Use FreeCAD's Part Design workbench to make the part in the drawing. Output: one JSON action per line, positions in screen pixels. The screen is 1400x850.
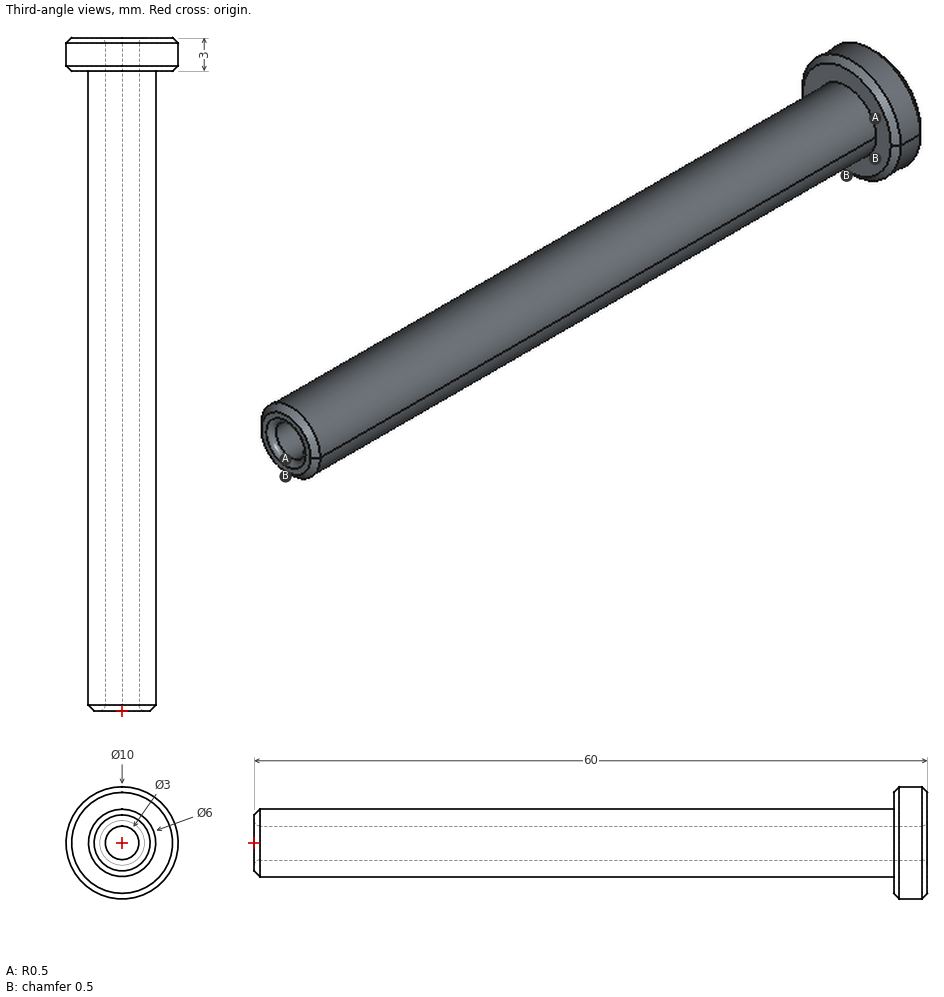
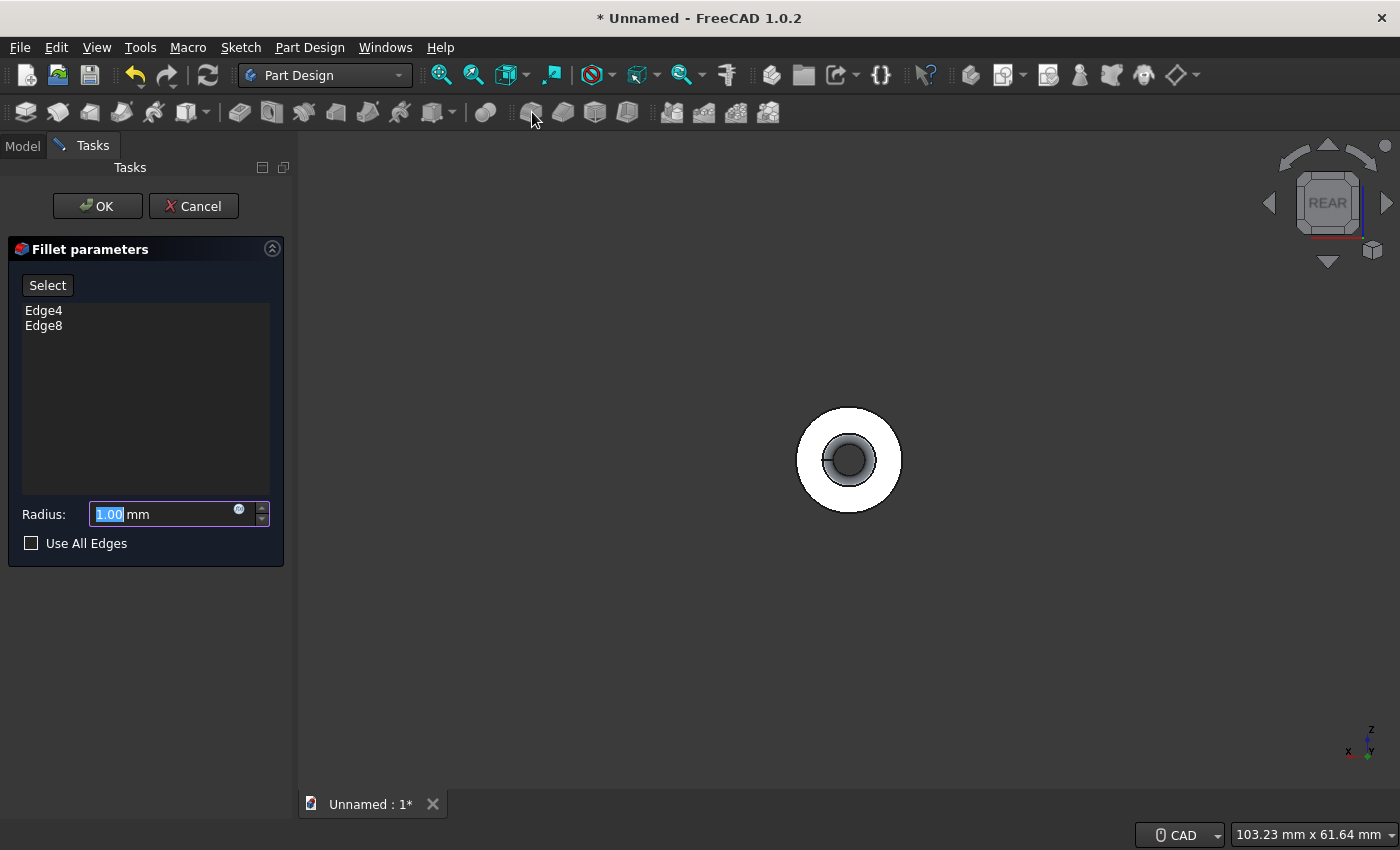
{"action": "type", "text": "0.5"}
{"action": "key", "text": "Tab"}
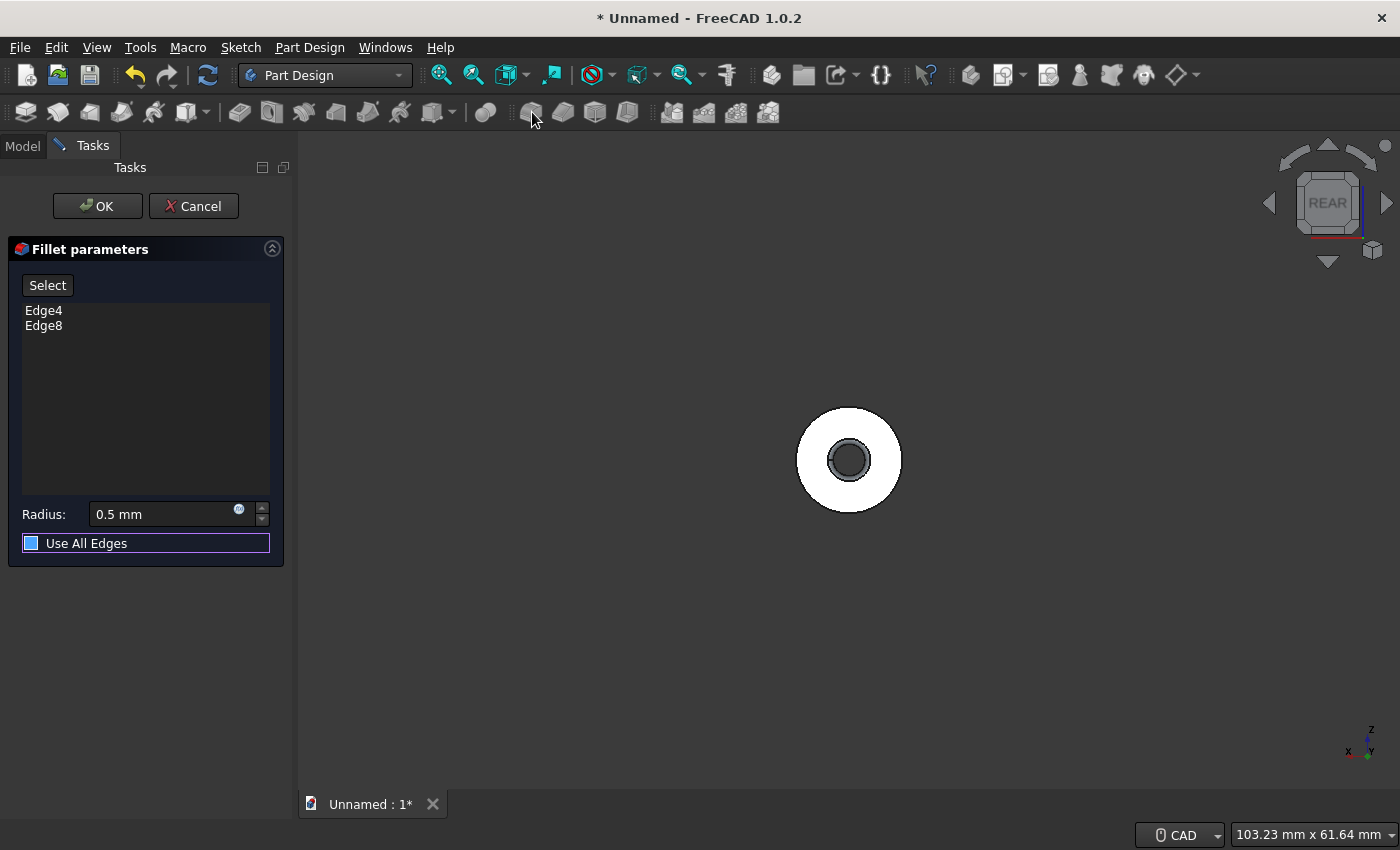
{"action": "left_click", "coordinate": [98, 206]}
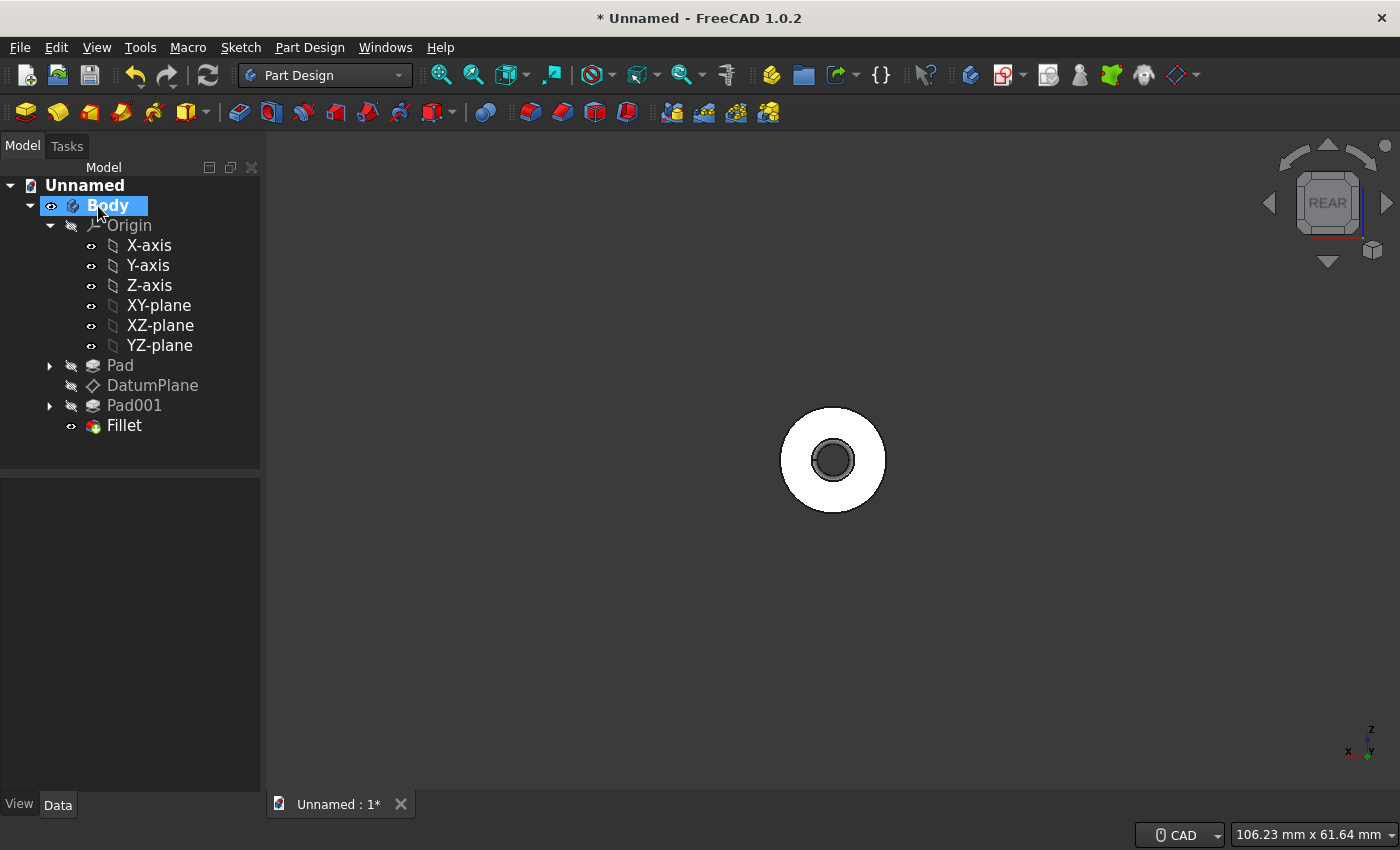
{"action": "left_click", "coordinate": [442, 76]}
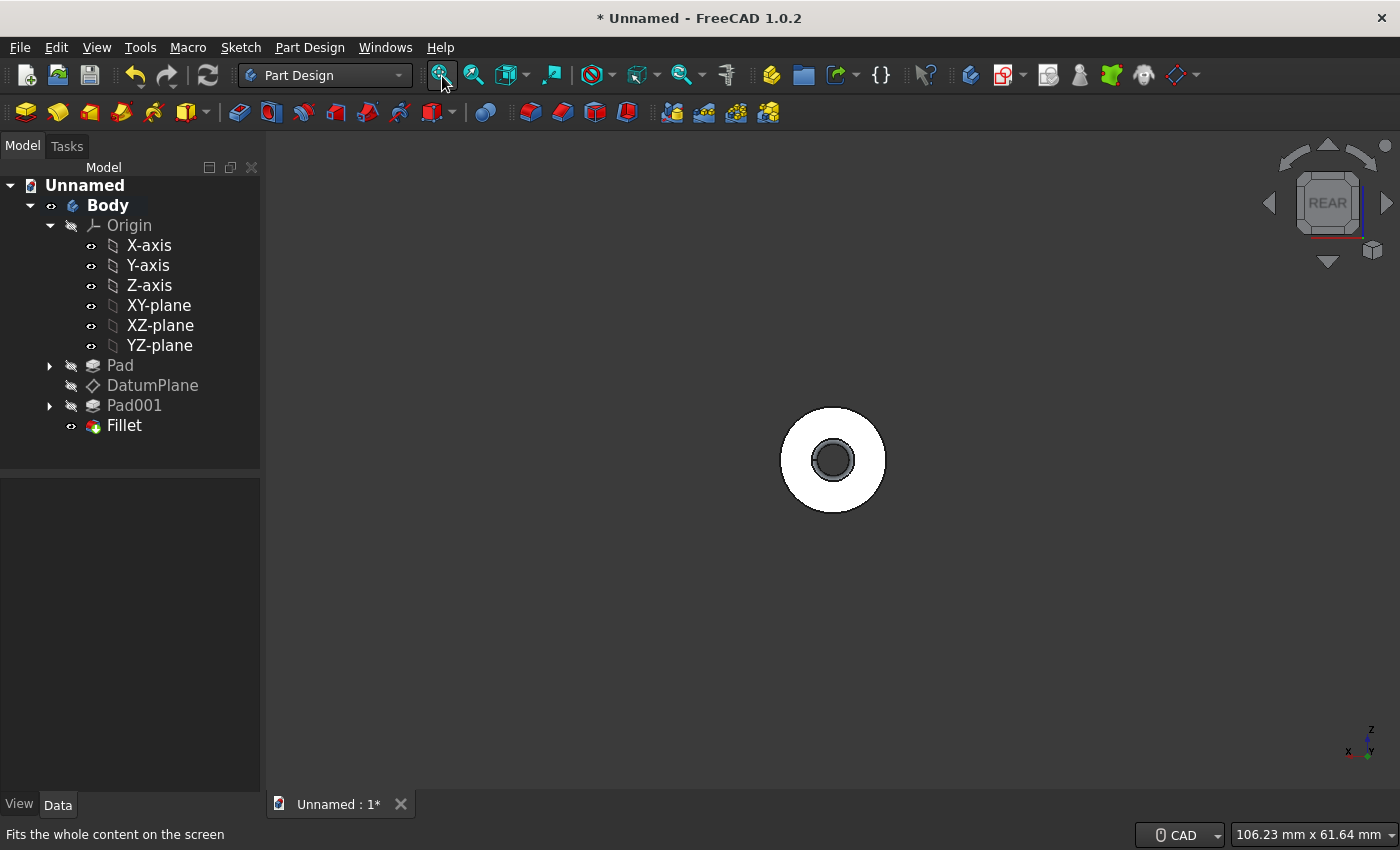
{"action": "left_click", "coordinate": [887, 459]}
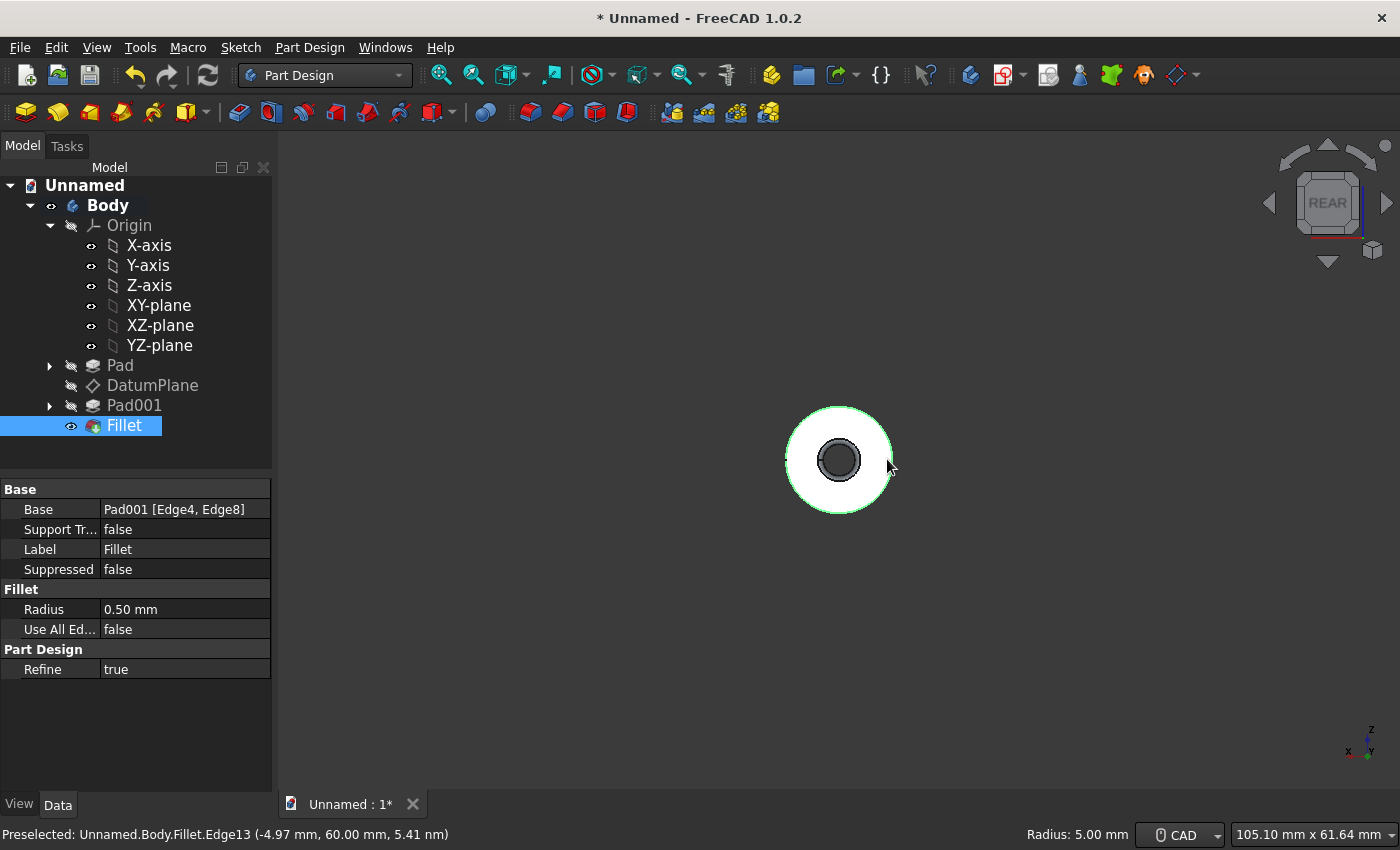
{"action": "key", "text": "0"}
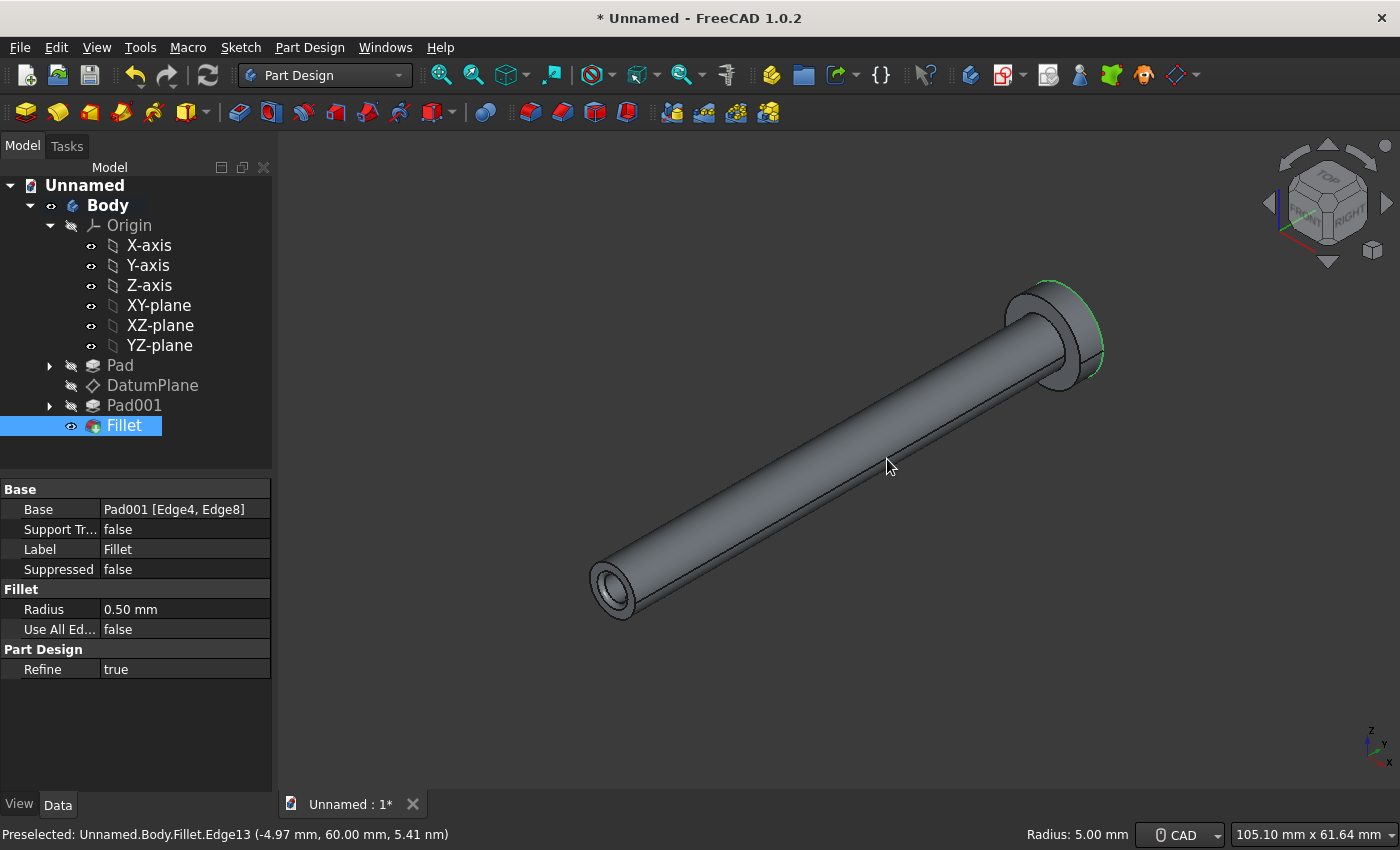
{"action": "left_click", "coordinate": [1012, 298], "text": "ctrl"}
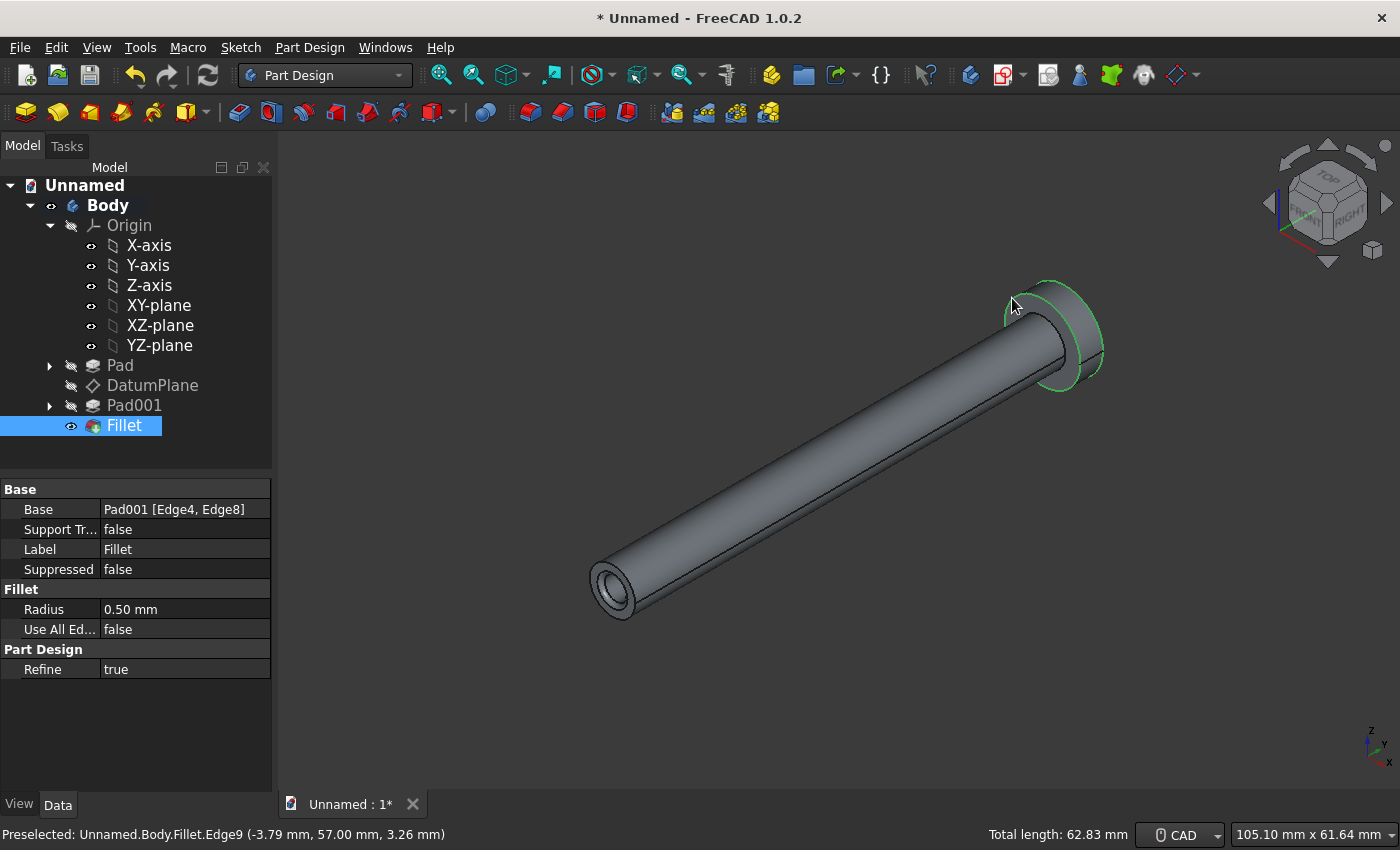
{"action": "left_click", "coordinate": [594, 564], "text": "ctrl"}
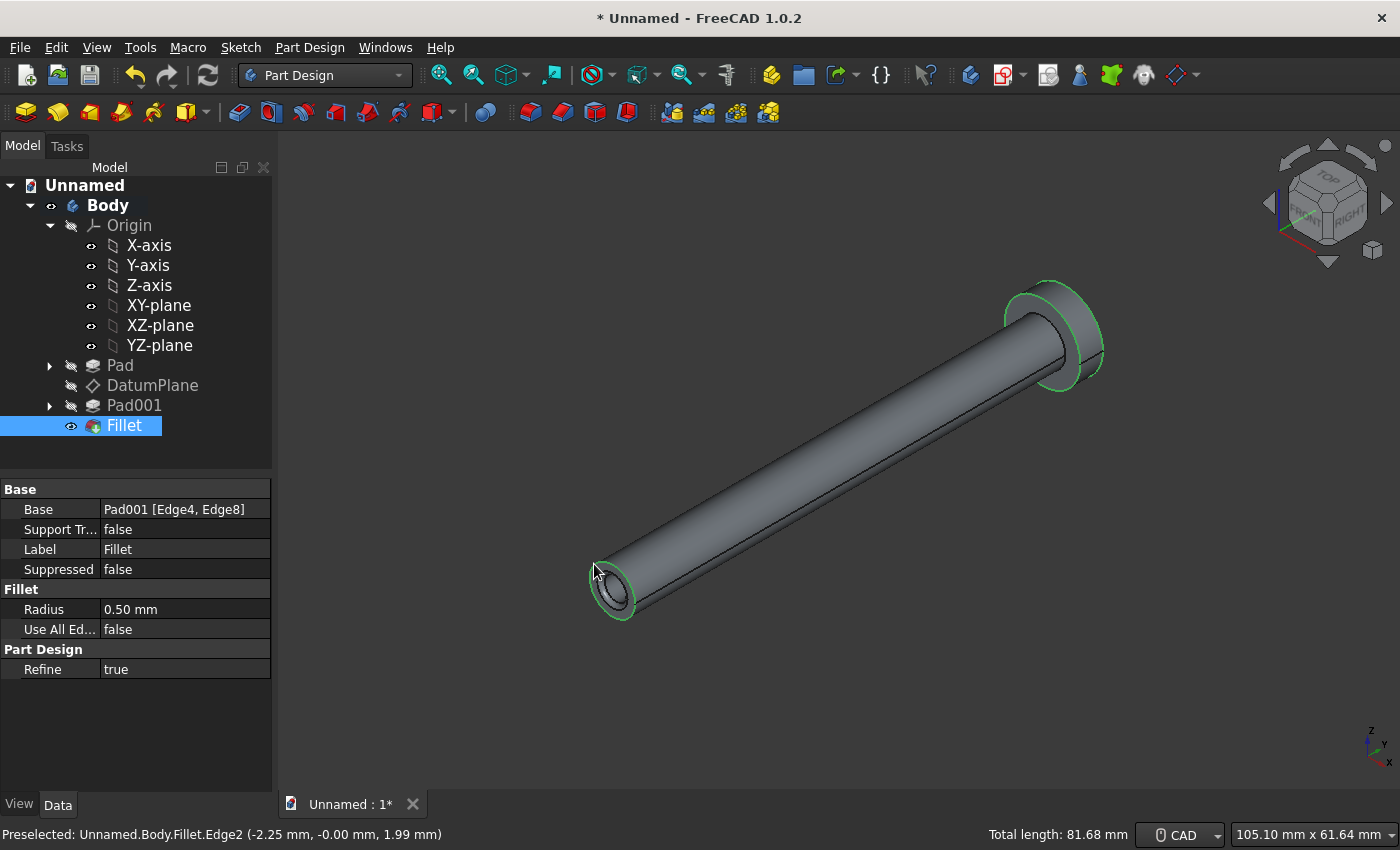
{"action": "left_click", "coordinate": [564, 112]}